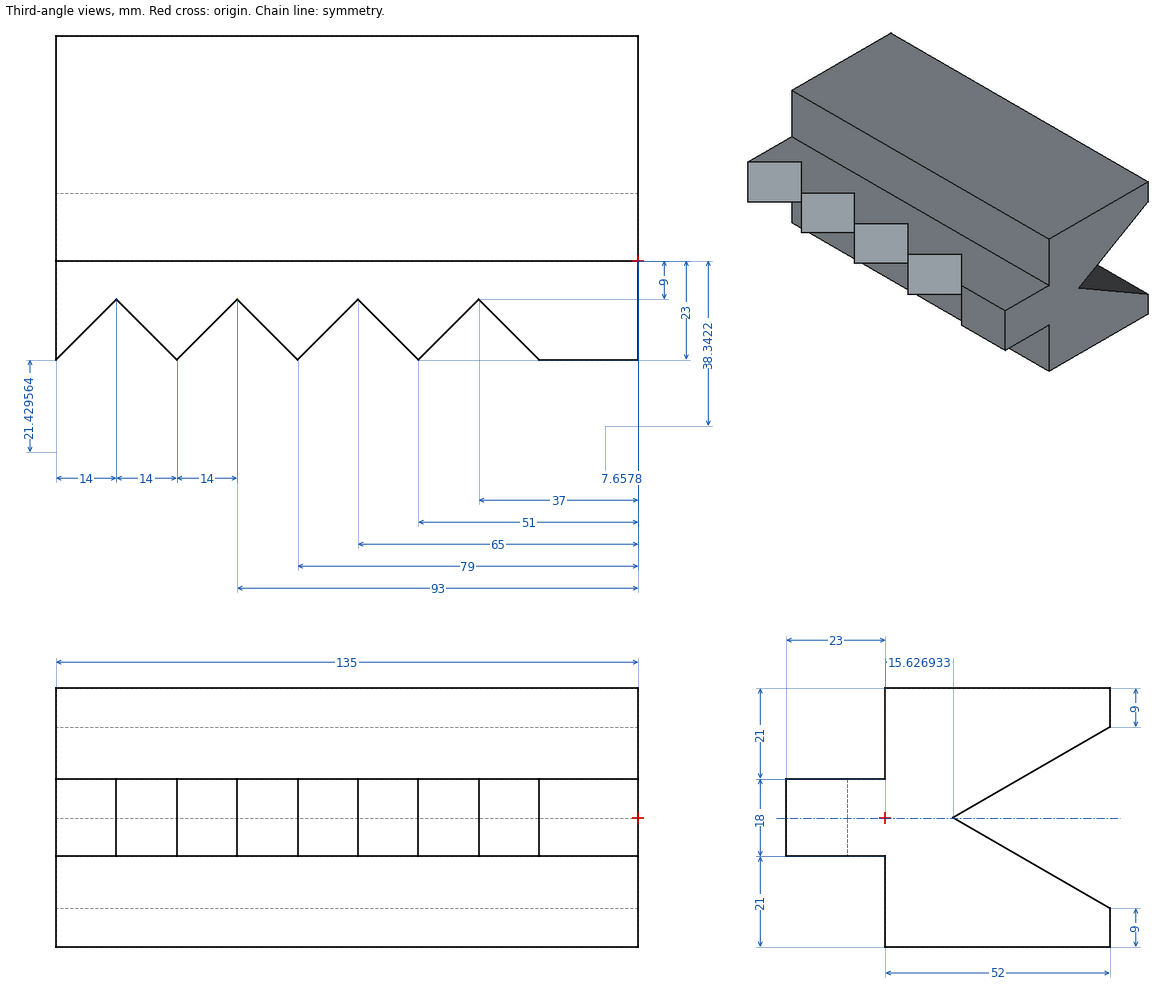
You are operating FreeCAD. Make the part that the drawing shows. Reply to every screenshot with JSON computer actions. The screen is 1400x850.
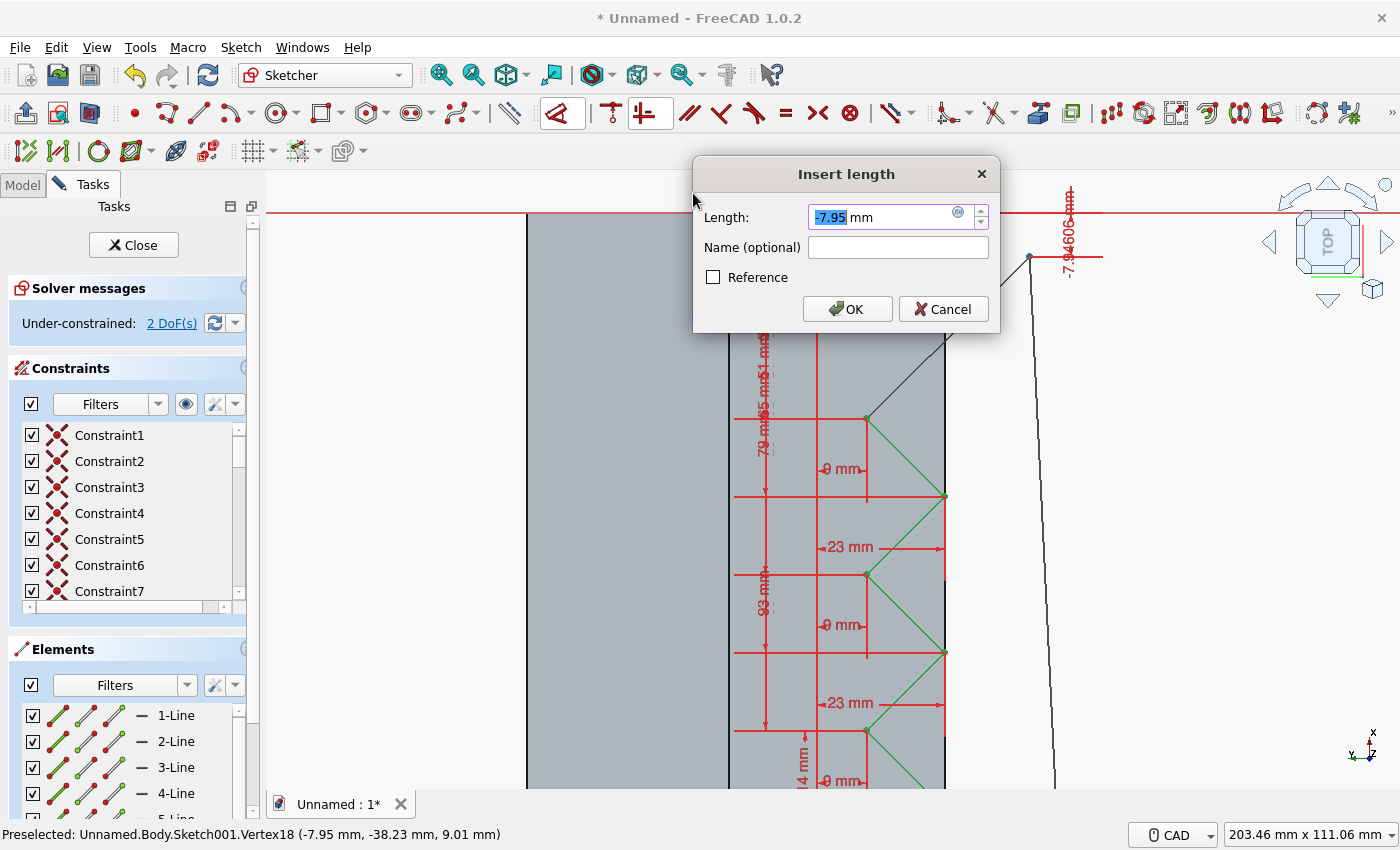
{"action": "type", "text": "-7.6578"}
{"action": "key", "text": "Return"}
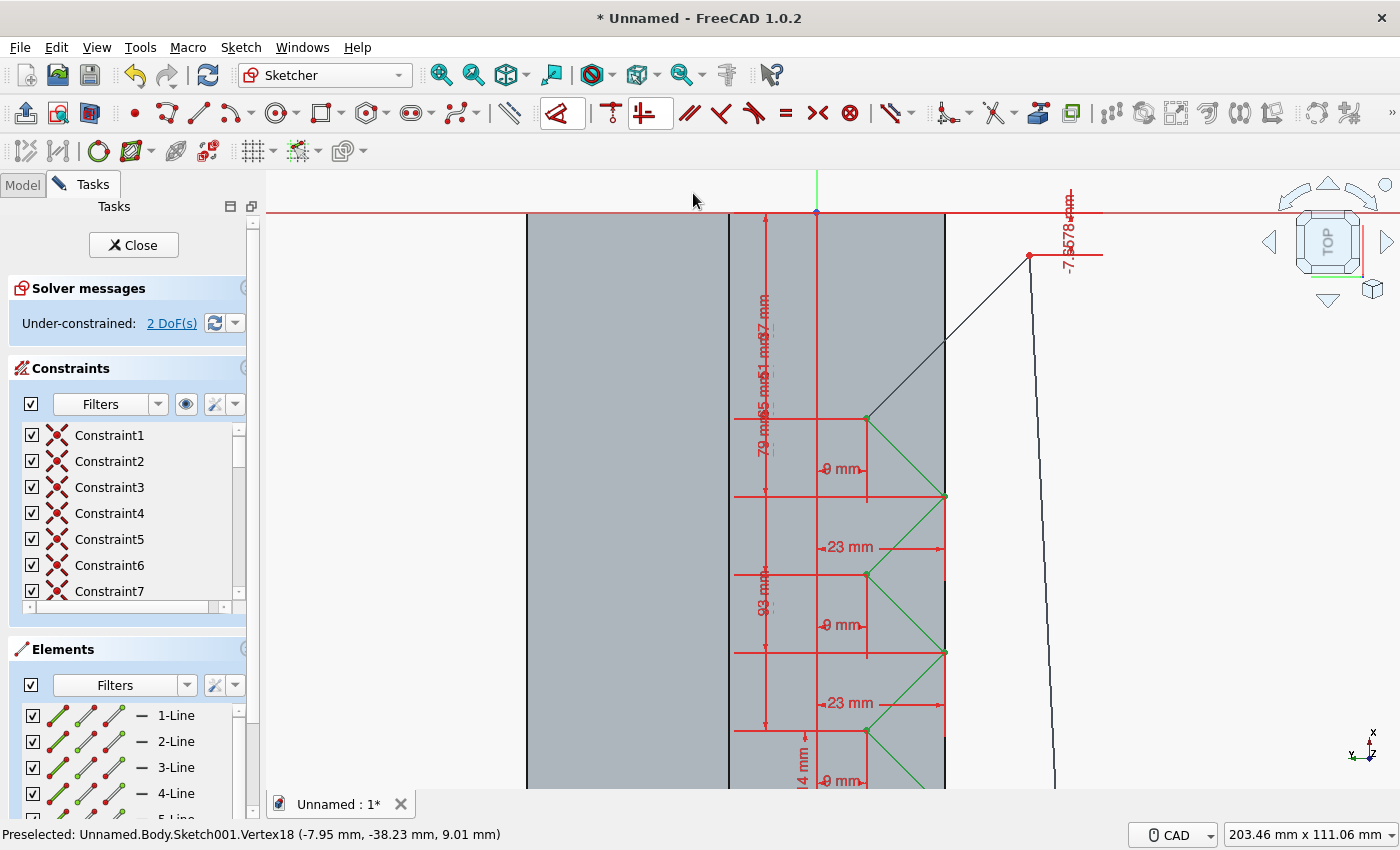
{"action": "left_click", "coordinate": [1030, 255]}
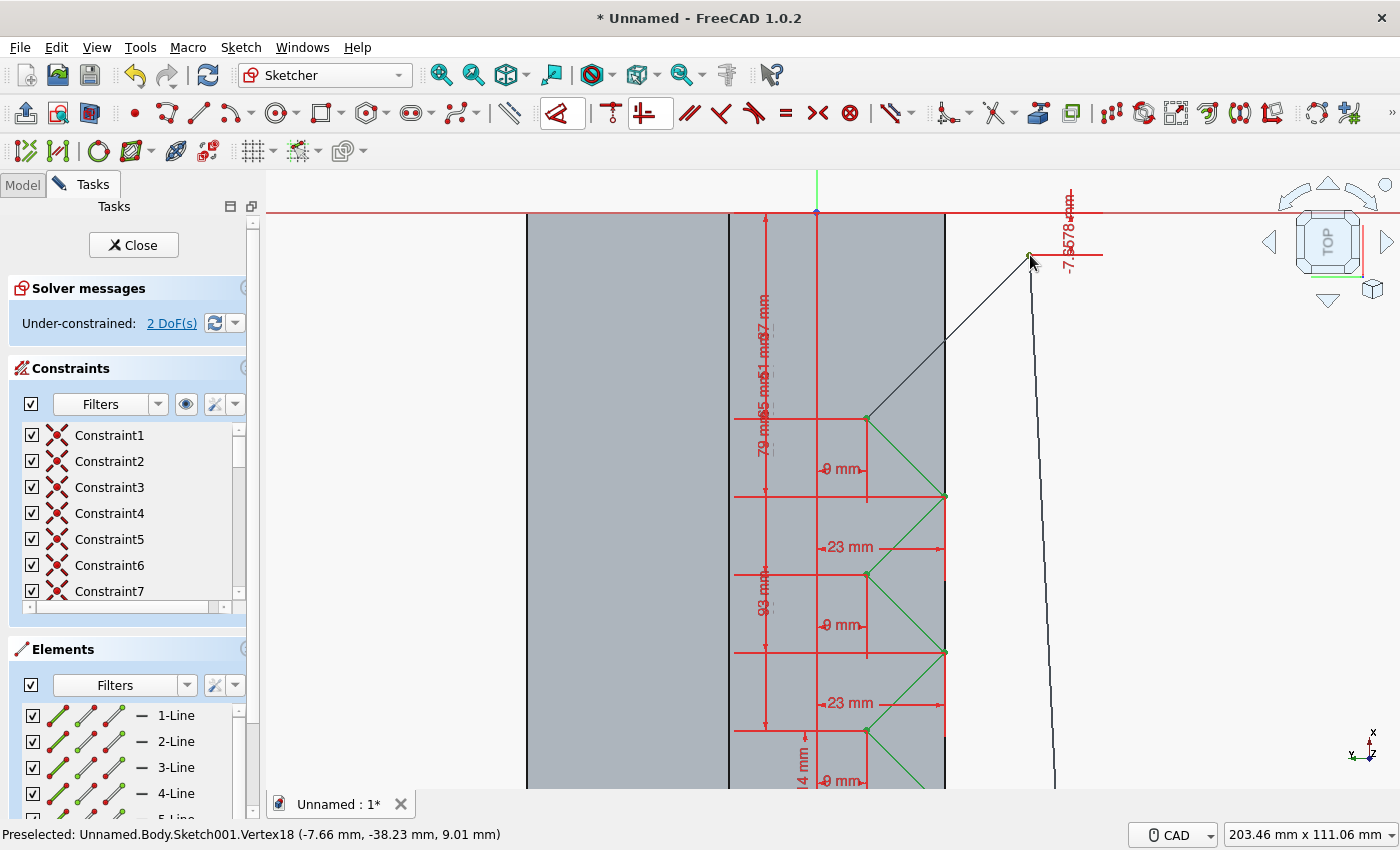
{"action": "key", "text": "l"}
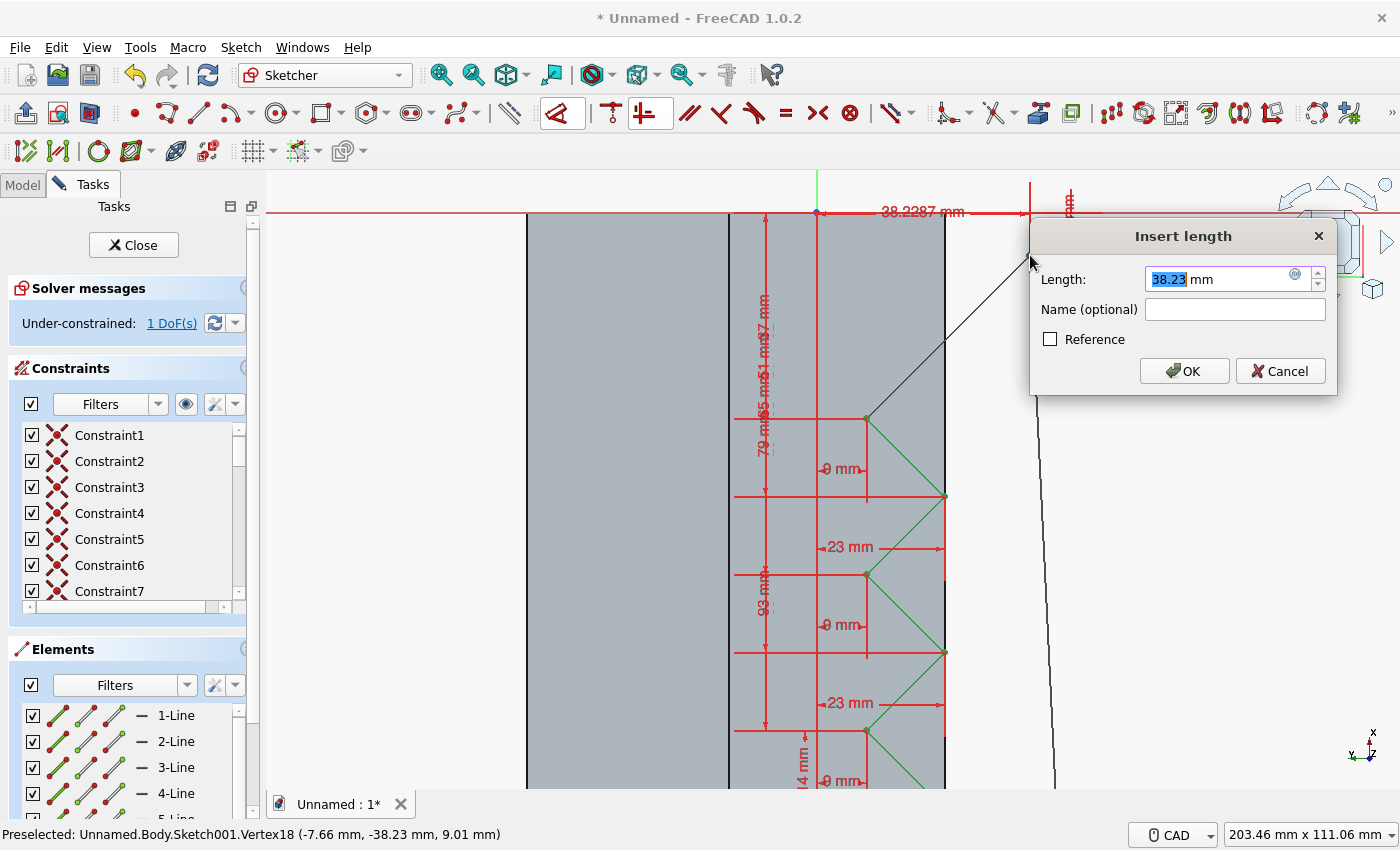
{"action": "type", "text": "38.3422"}
{"action": "key", "text": "Return"}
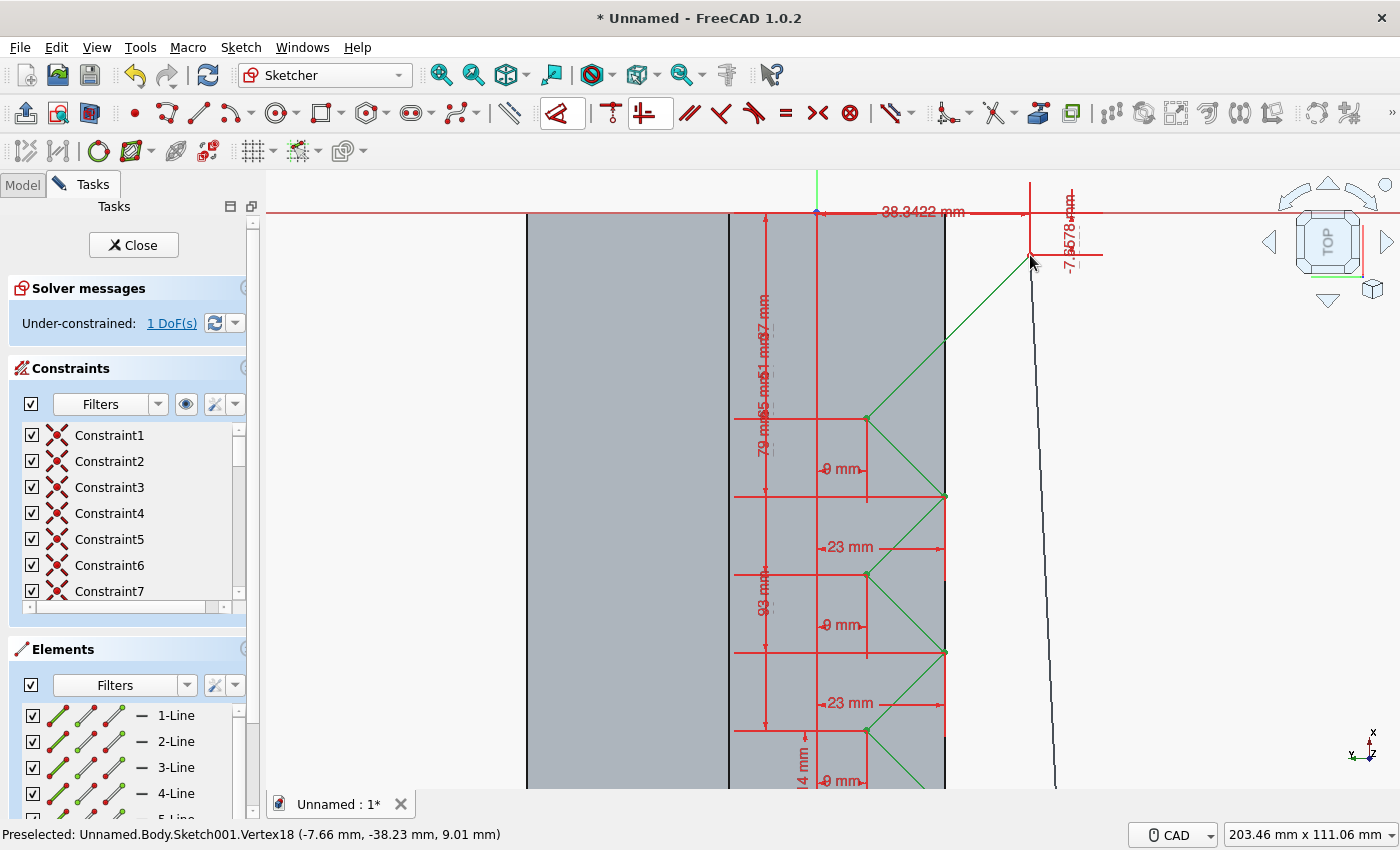
{"action": "scroll", "coordinate": [551, 346], "scroll_direction": "down", "scroll_amount": 3}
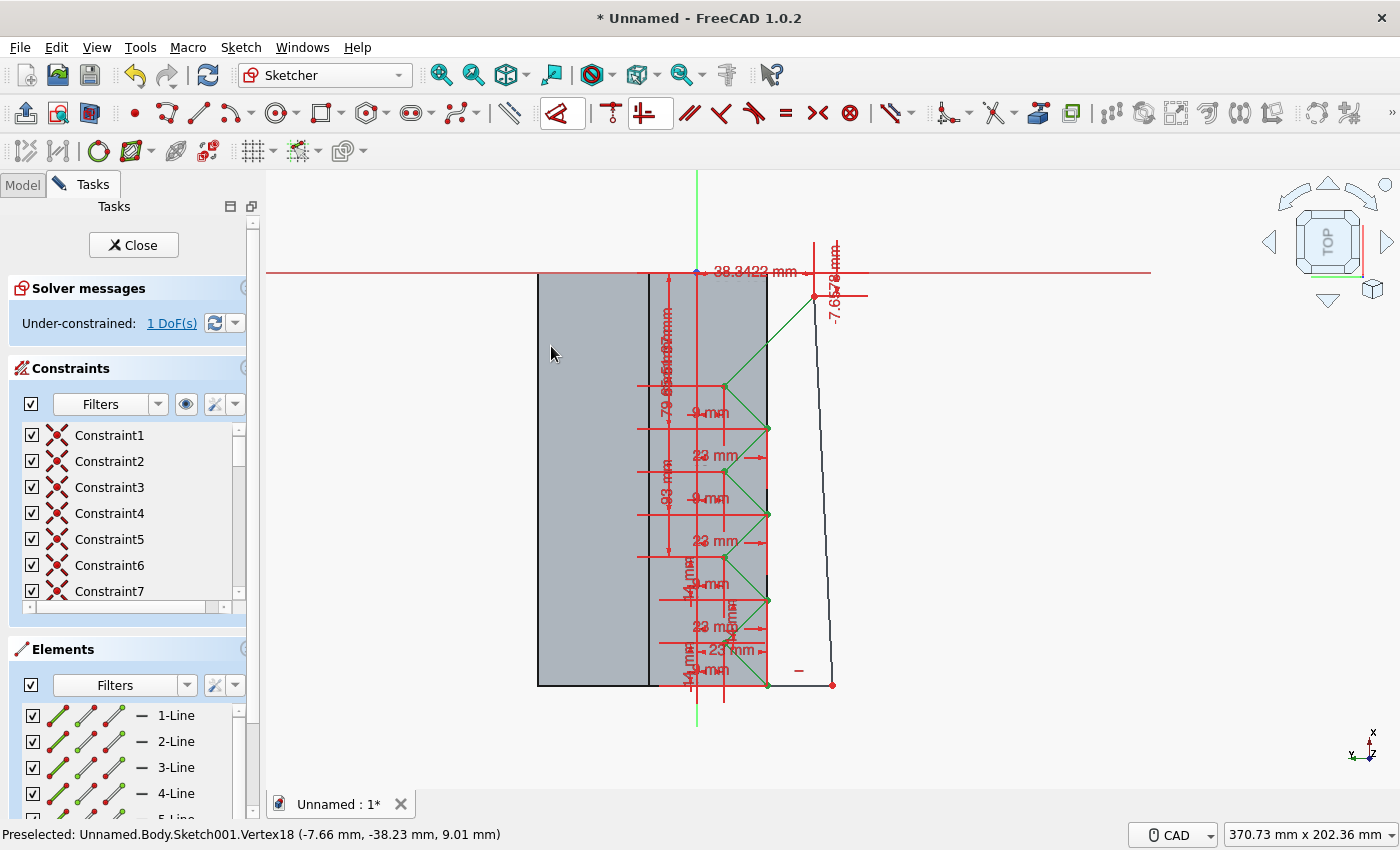
{"action": "left_click", "coordinate": [787, 686]}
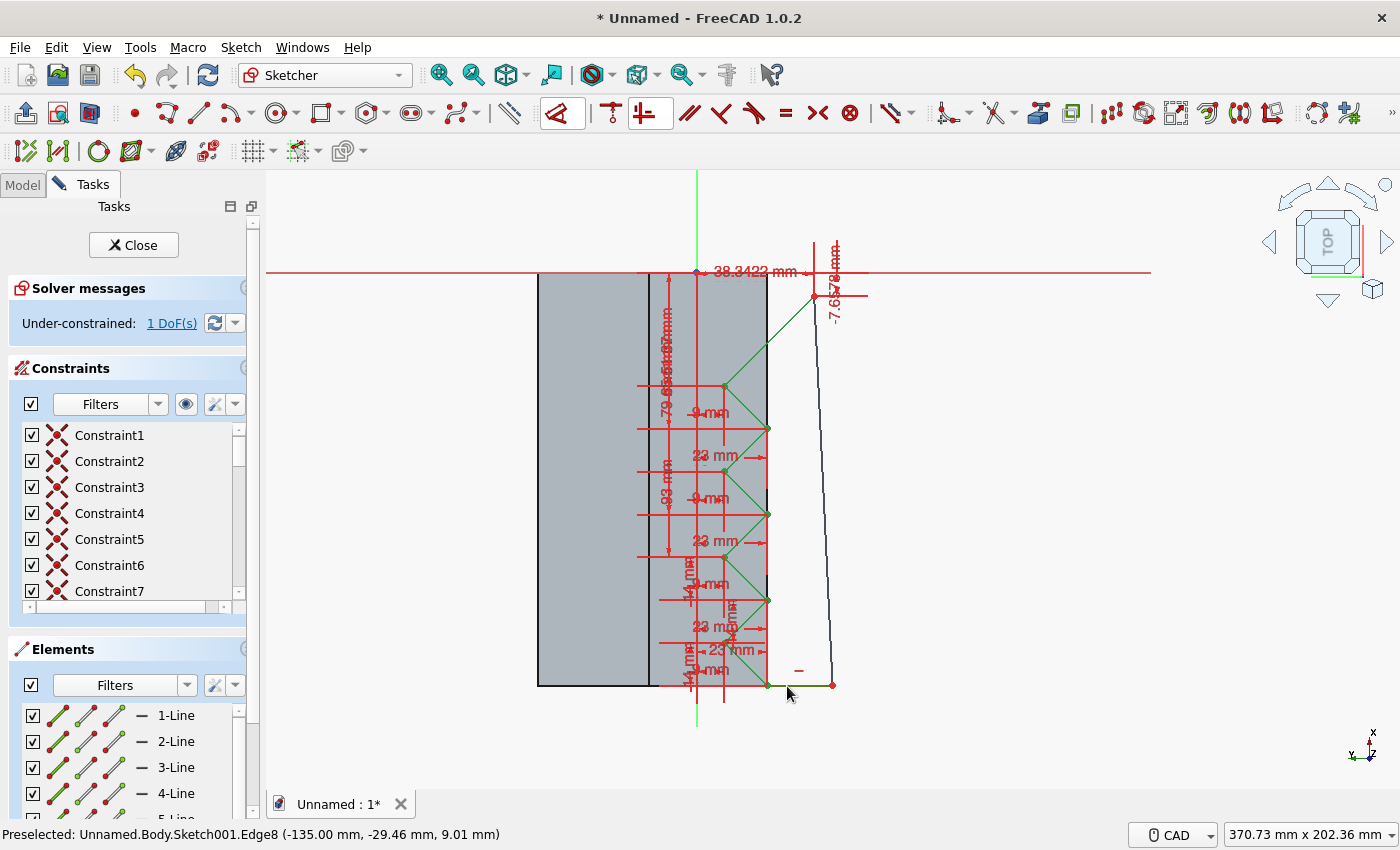
{"action": "key", "text": "l"}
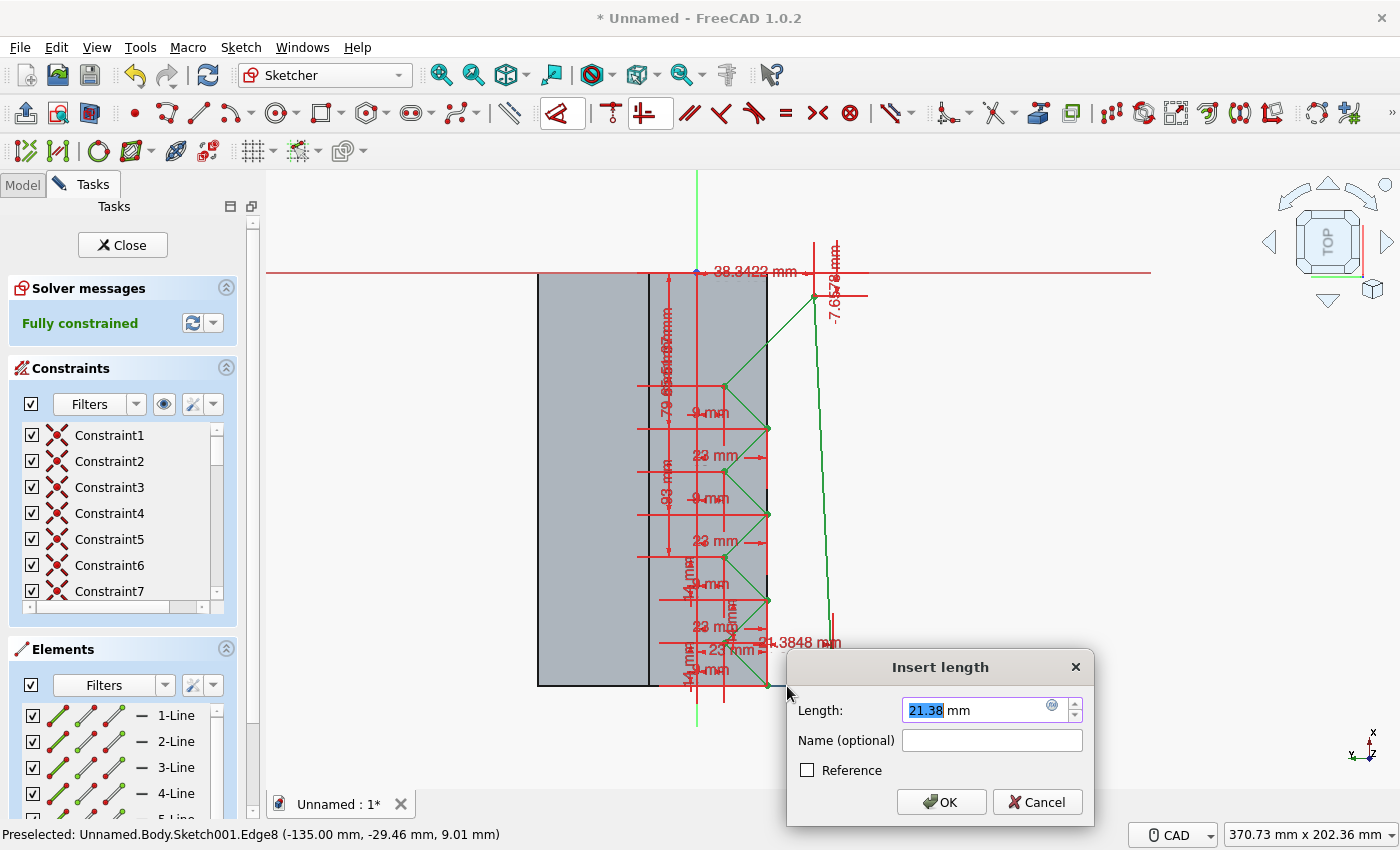
{"action": "type", "text": "21.429564"}
{"action": "key", "text": "Return"}